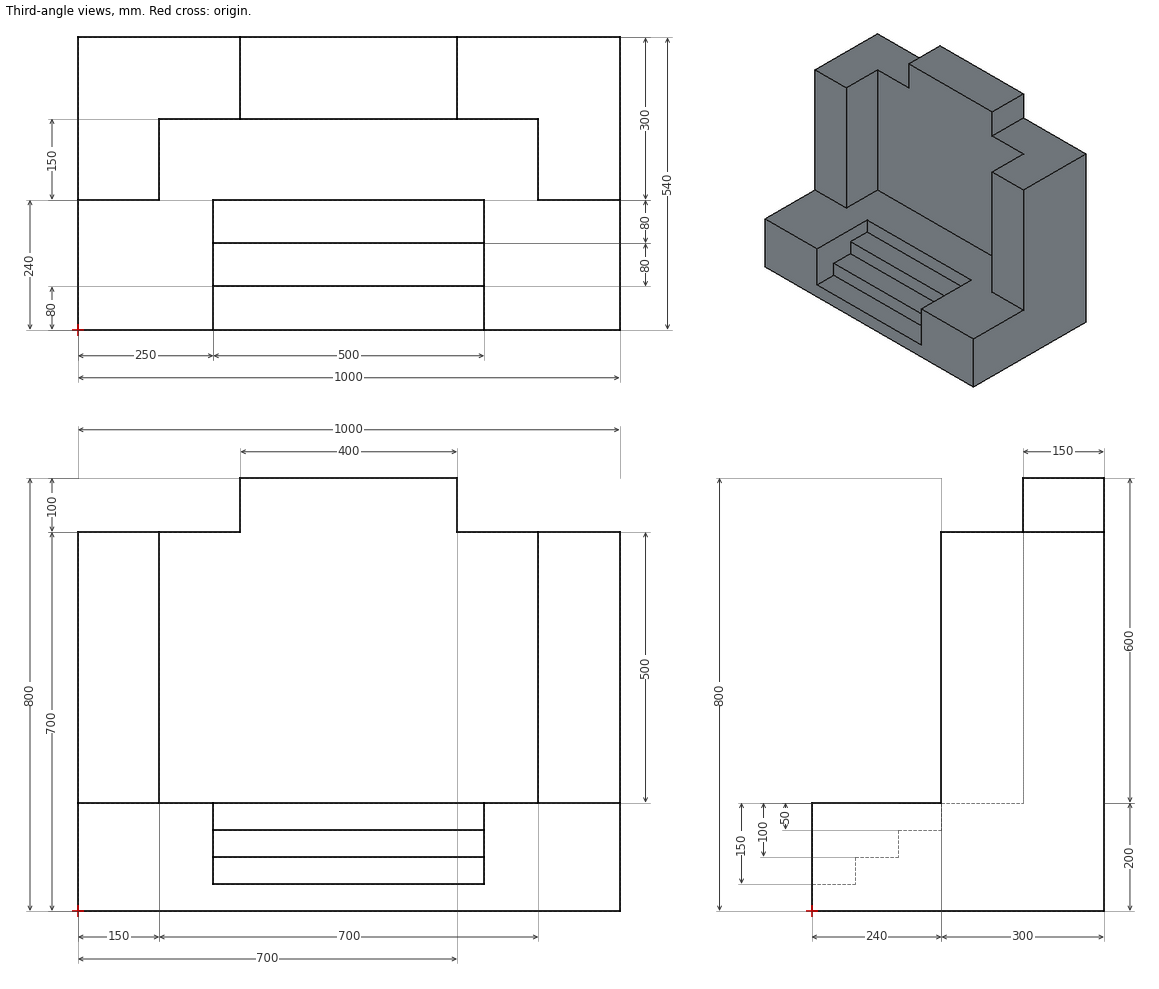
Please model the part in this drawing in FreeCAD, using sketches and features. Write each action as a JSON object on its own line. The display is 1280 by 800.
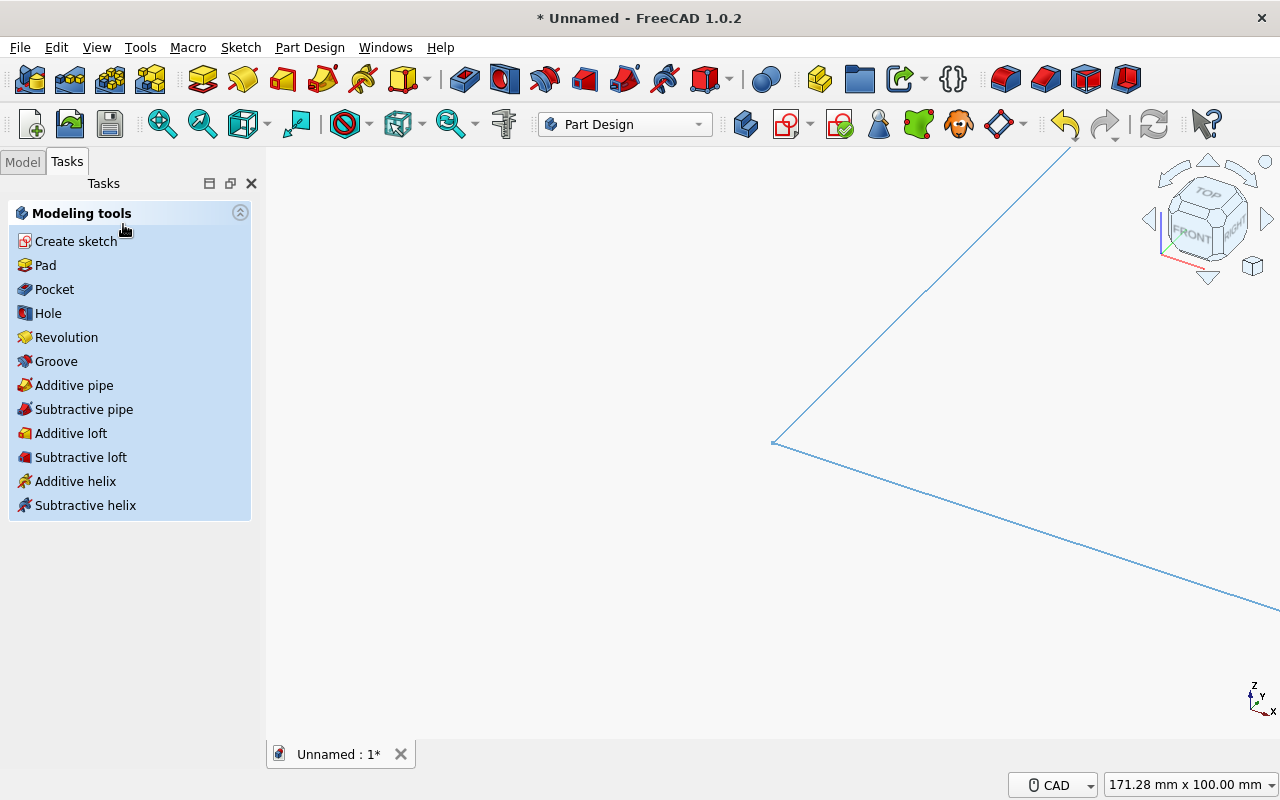
{"action": "left_click", "coordinate": [204, 80]}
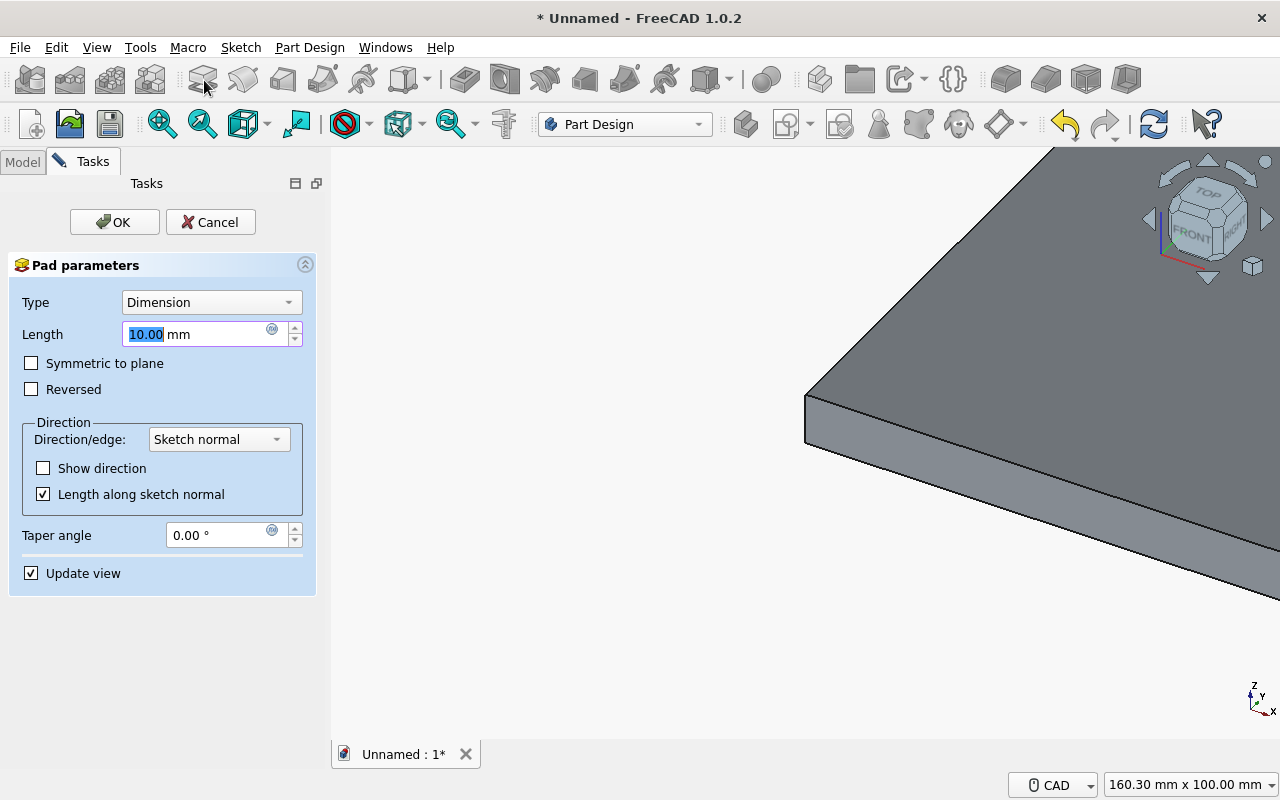
{"action": "type", "text": "200"}
{"action": "key", "text": "Tab"}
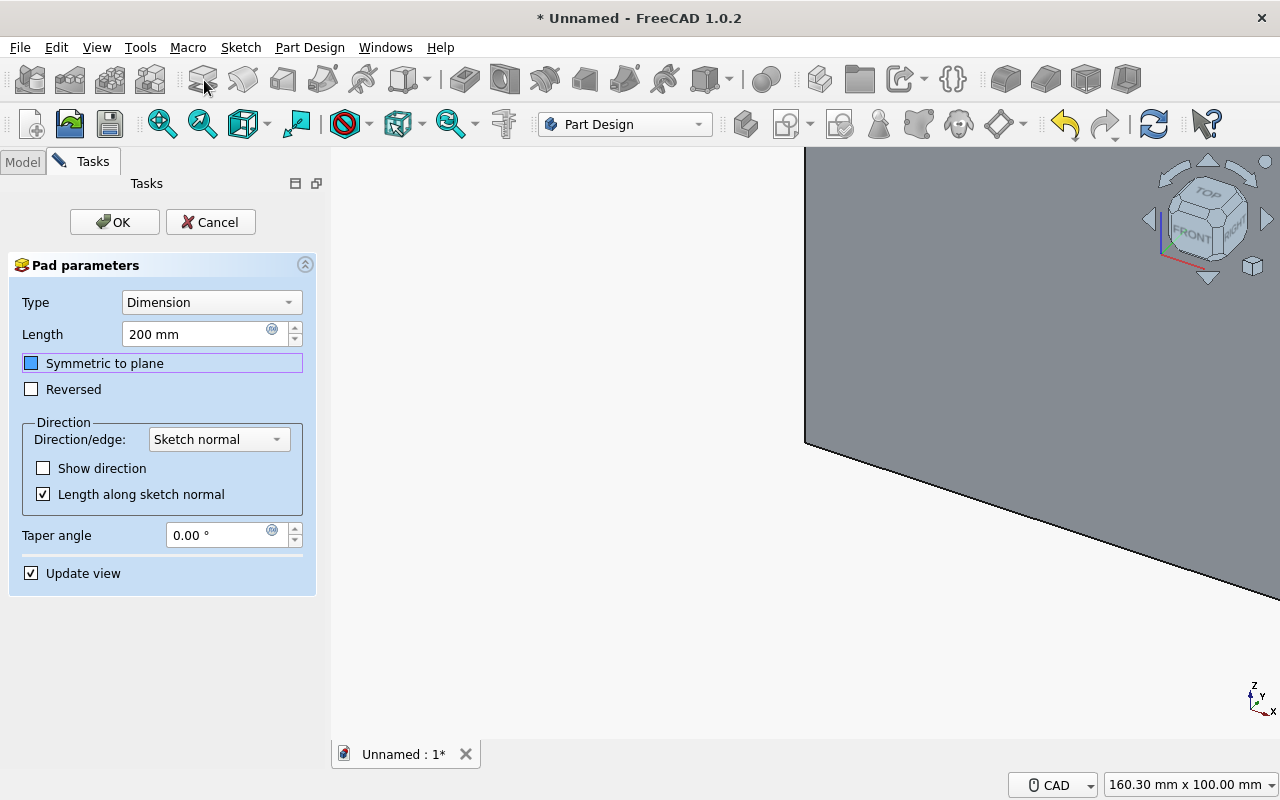
{"action": "left_click", "coordinate": [115, 222]}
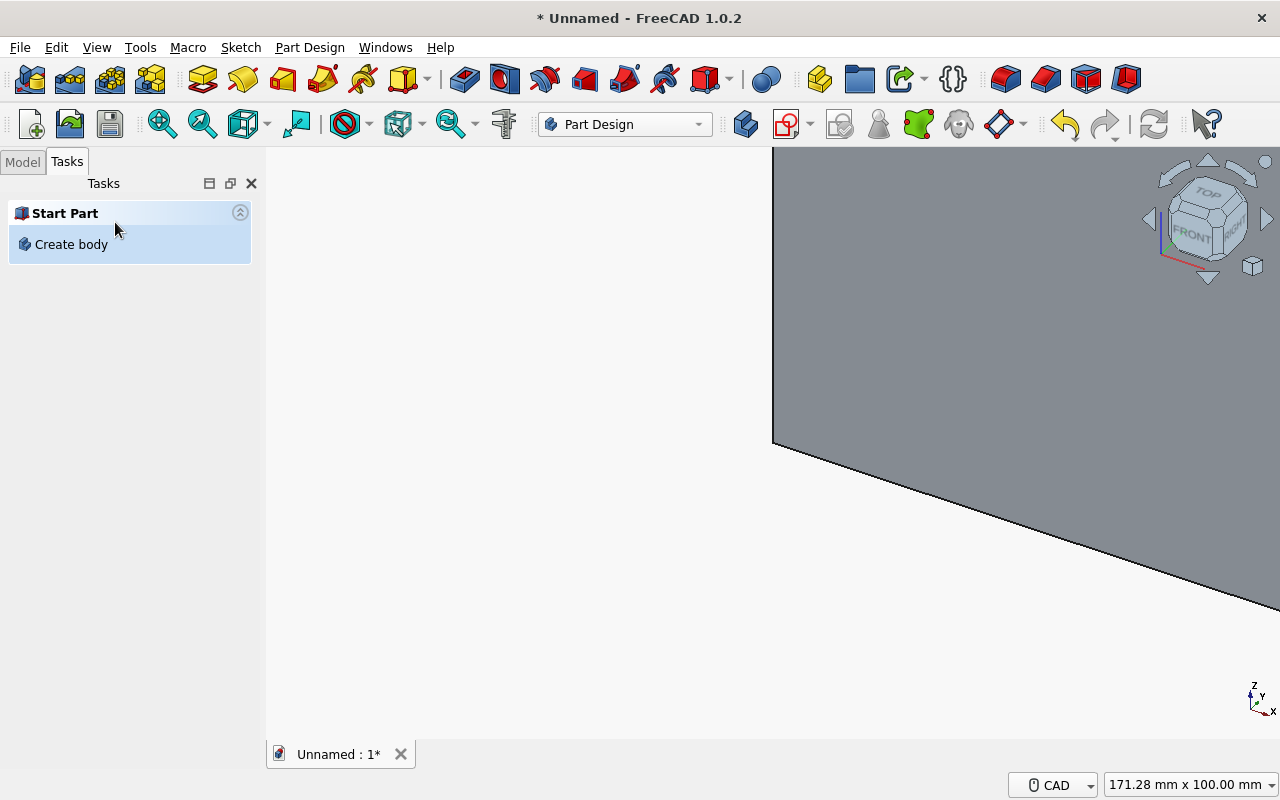
{"action": "left_click", "coordinate": [164, 124]}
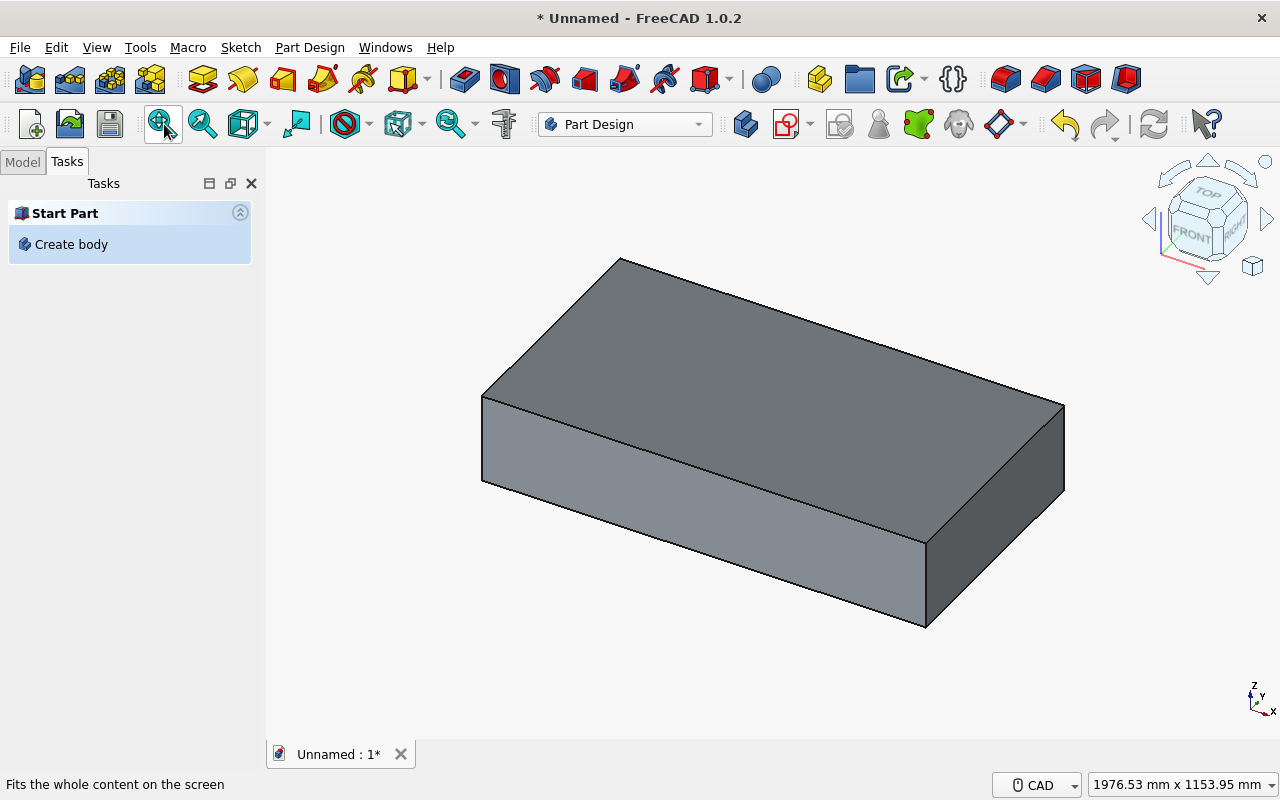
{"action": "left_click", "coordinate": [1035, 476]}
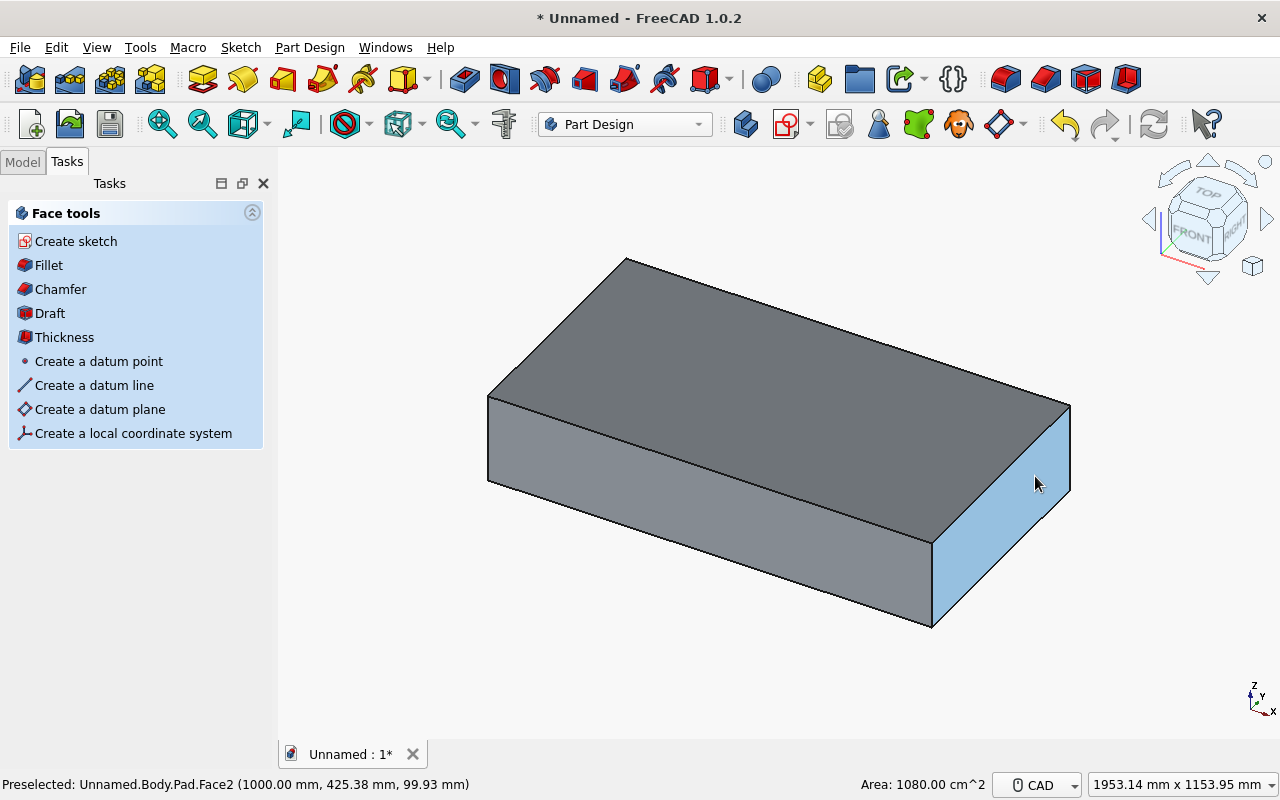
{"action": "left_click", "coordinate": [786, 124]}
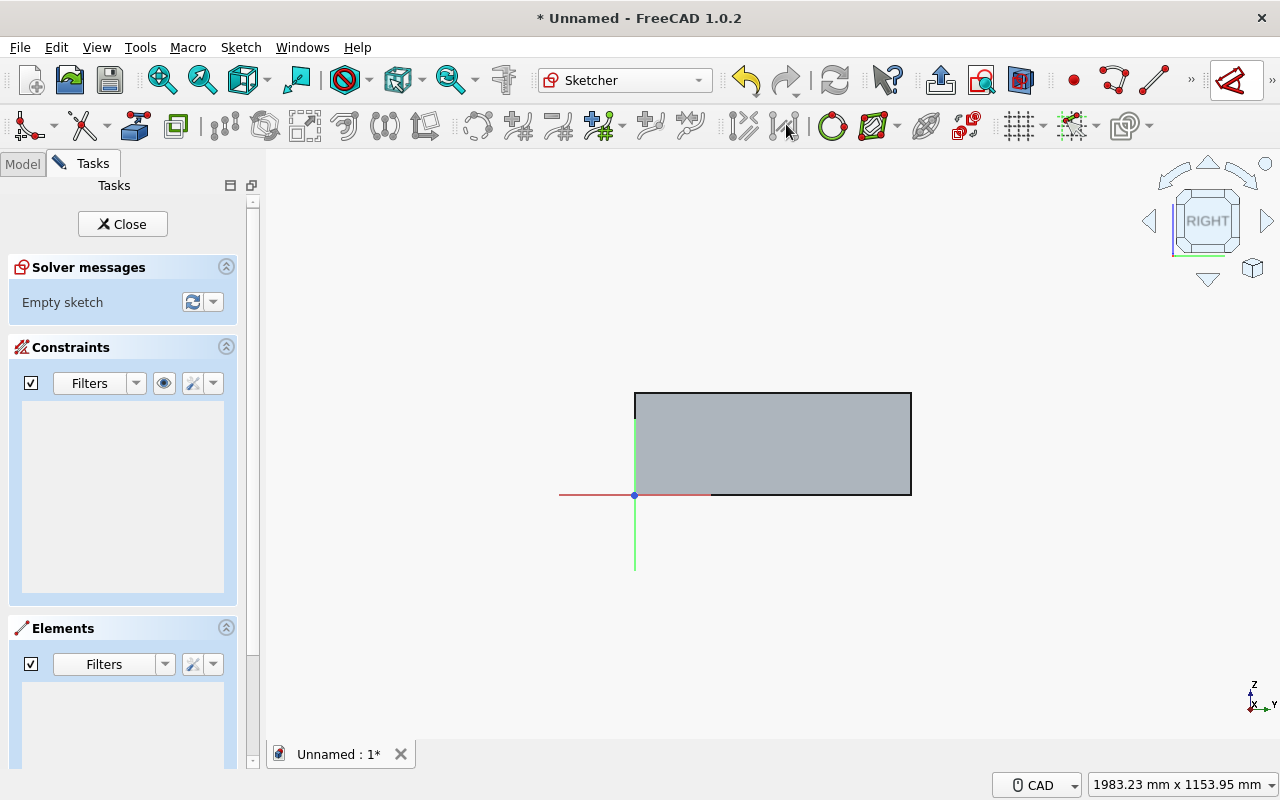
{"action": "scroll", "coordinate": [565, 711], "scroll_direction": "down", "scroll_amount": 2}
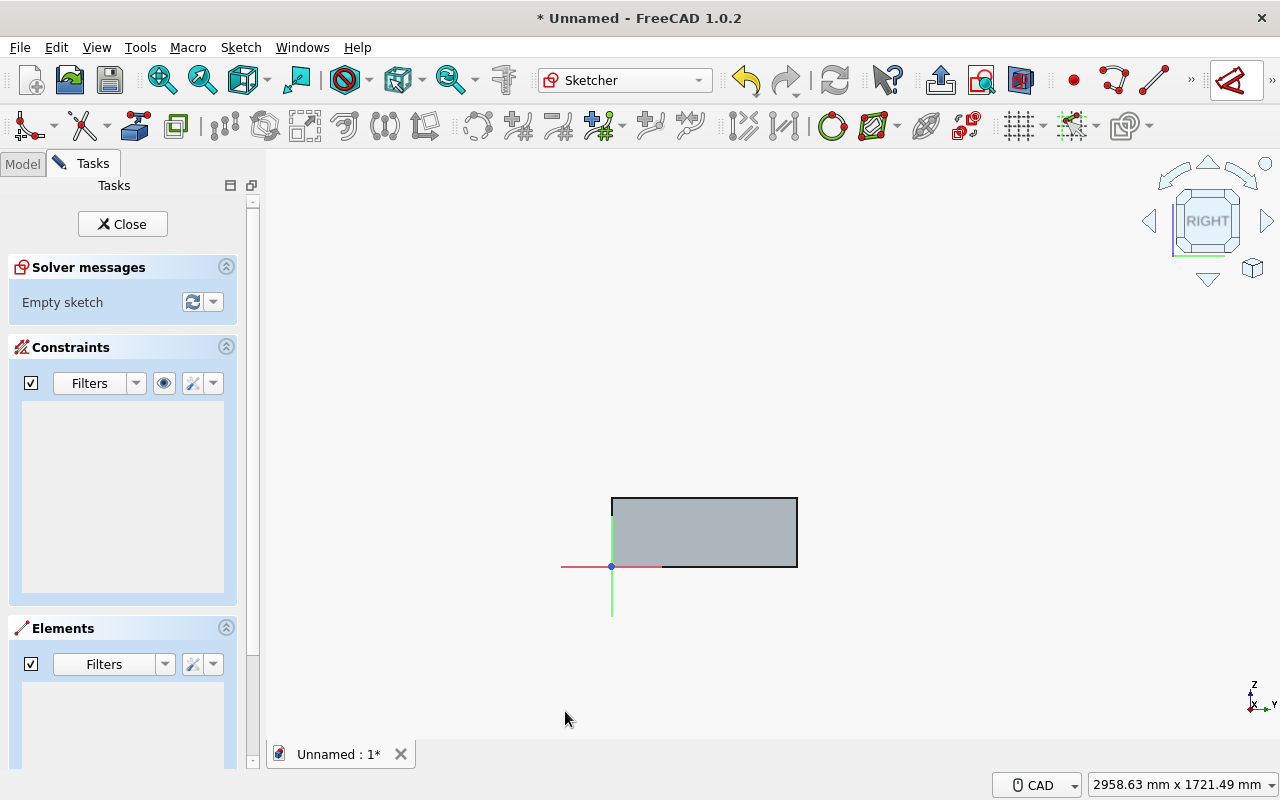
{"action": "scroll", "coordinate": [705, 400], "scroll_direction": "up", "scroll_amount": 2}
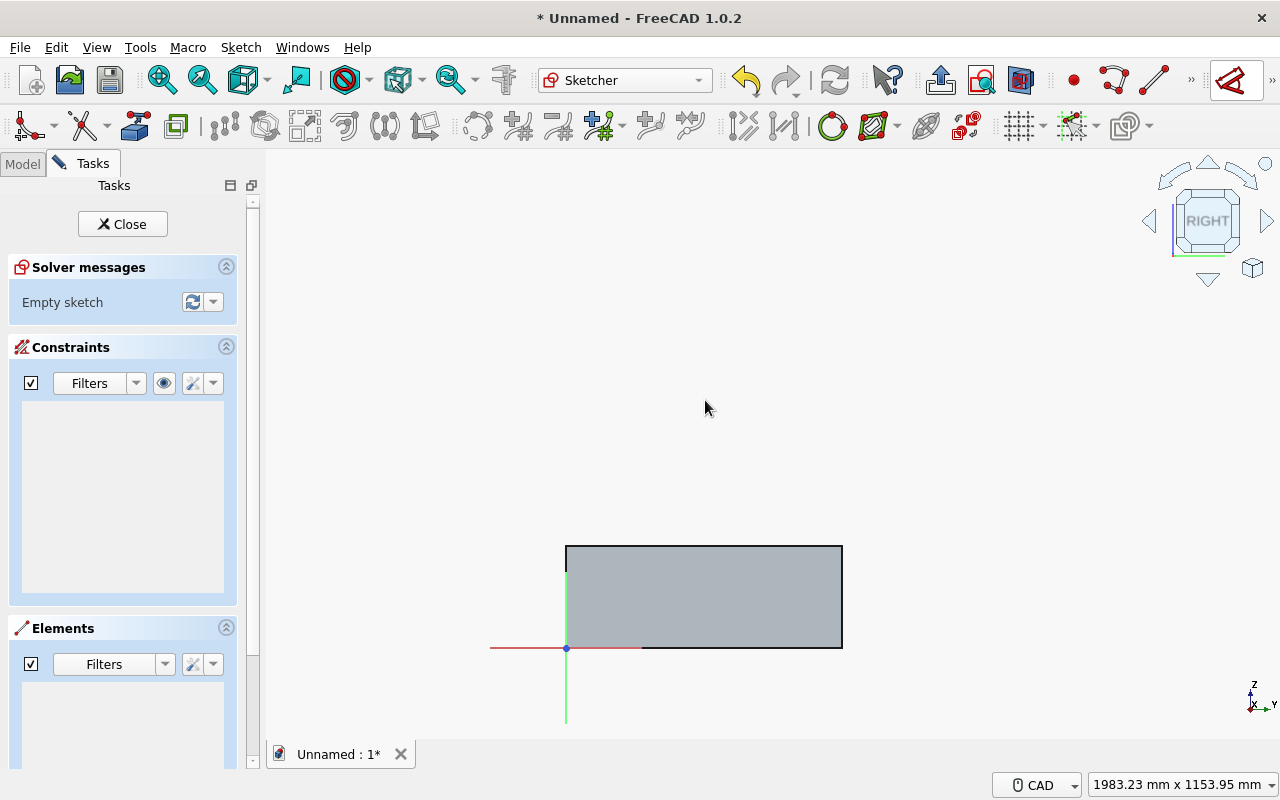
{"action": "key", "text": "g r"}